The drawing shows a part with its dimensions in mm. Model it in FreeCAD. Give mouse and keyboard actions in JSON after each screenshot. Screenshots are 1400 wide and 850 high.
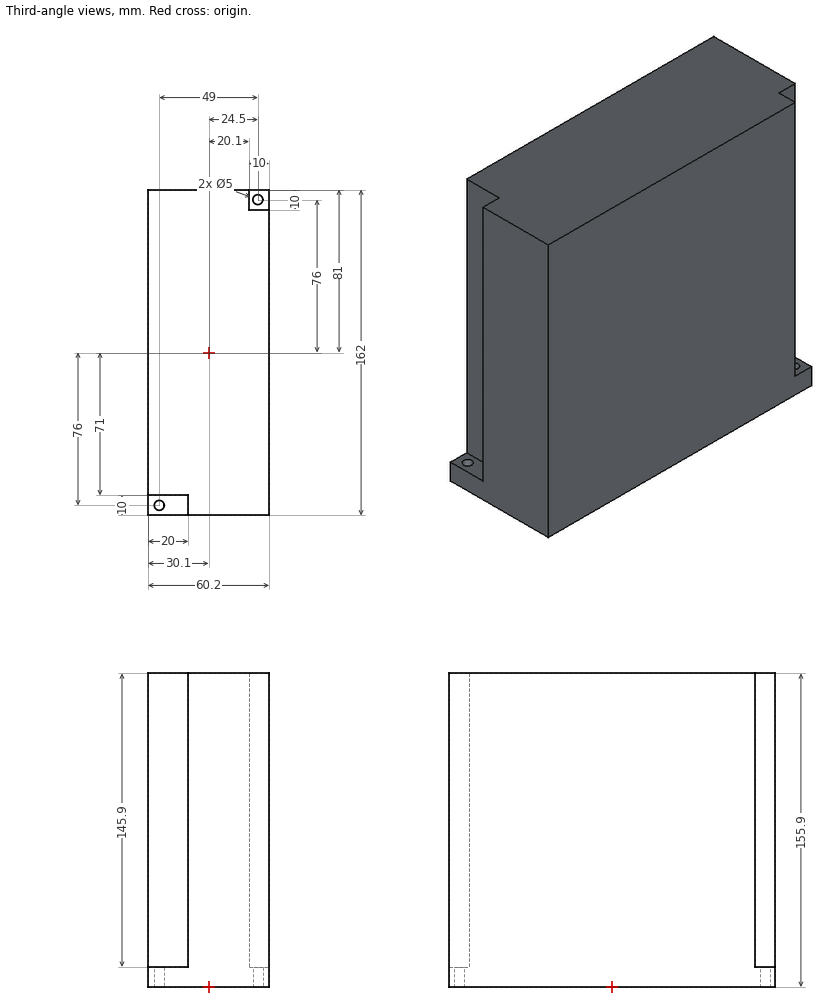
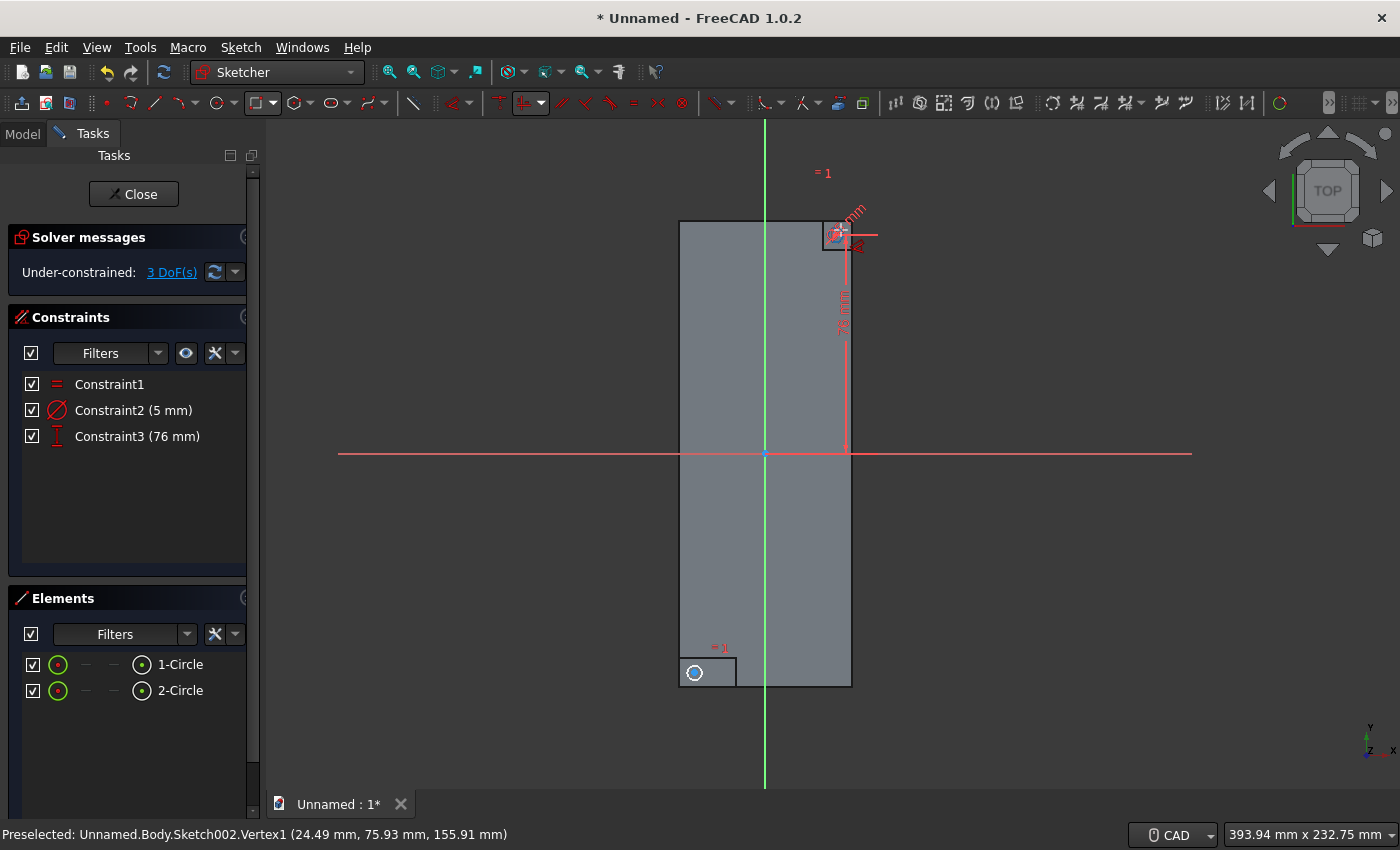
{"action": "left_click", "coordinate": [695, 673]}
{"action": "left_click", "coordinate": [661, 563]}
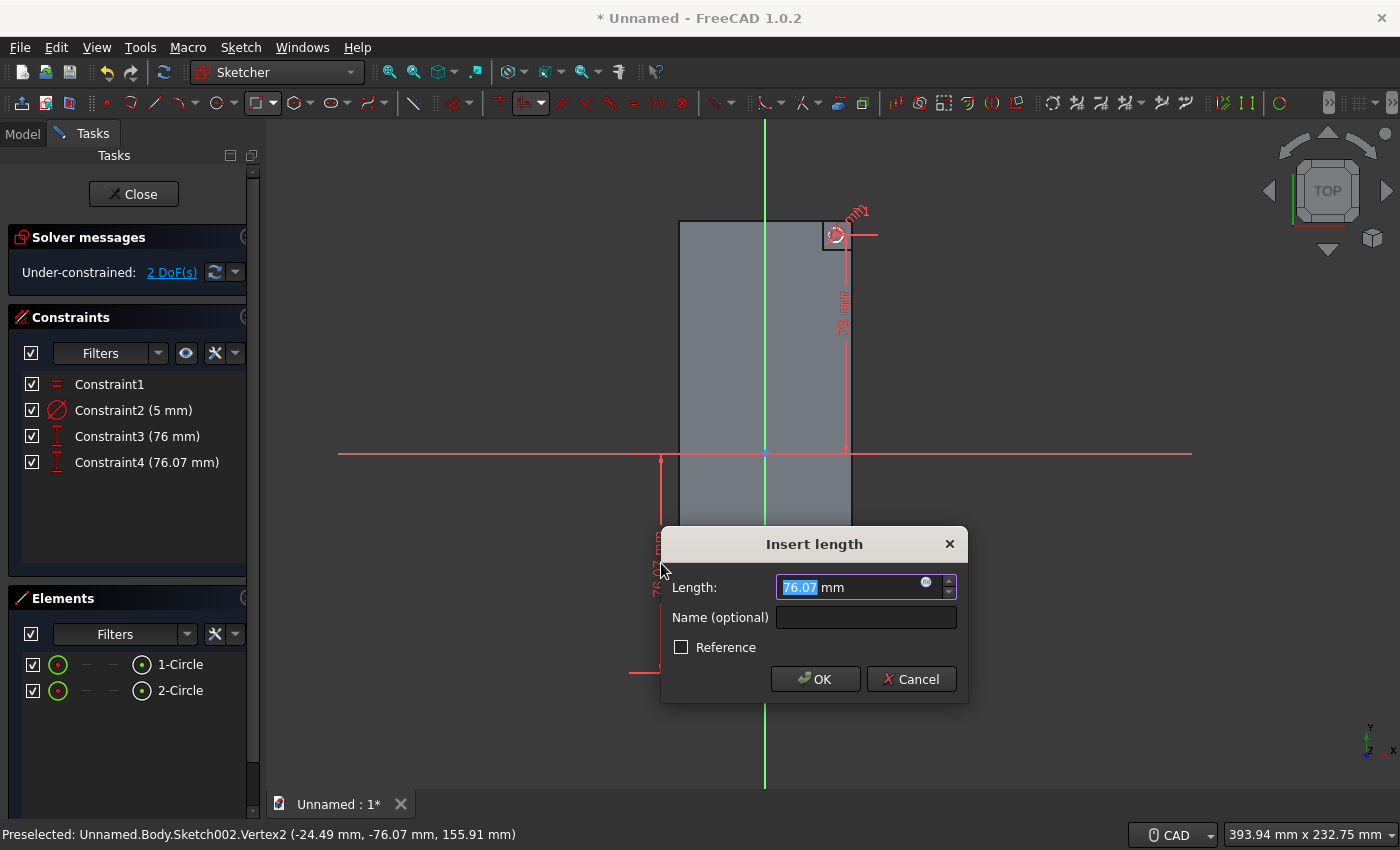
{"action": "type", "text": "76"}
{"action": "key", "text": "Return"}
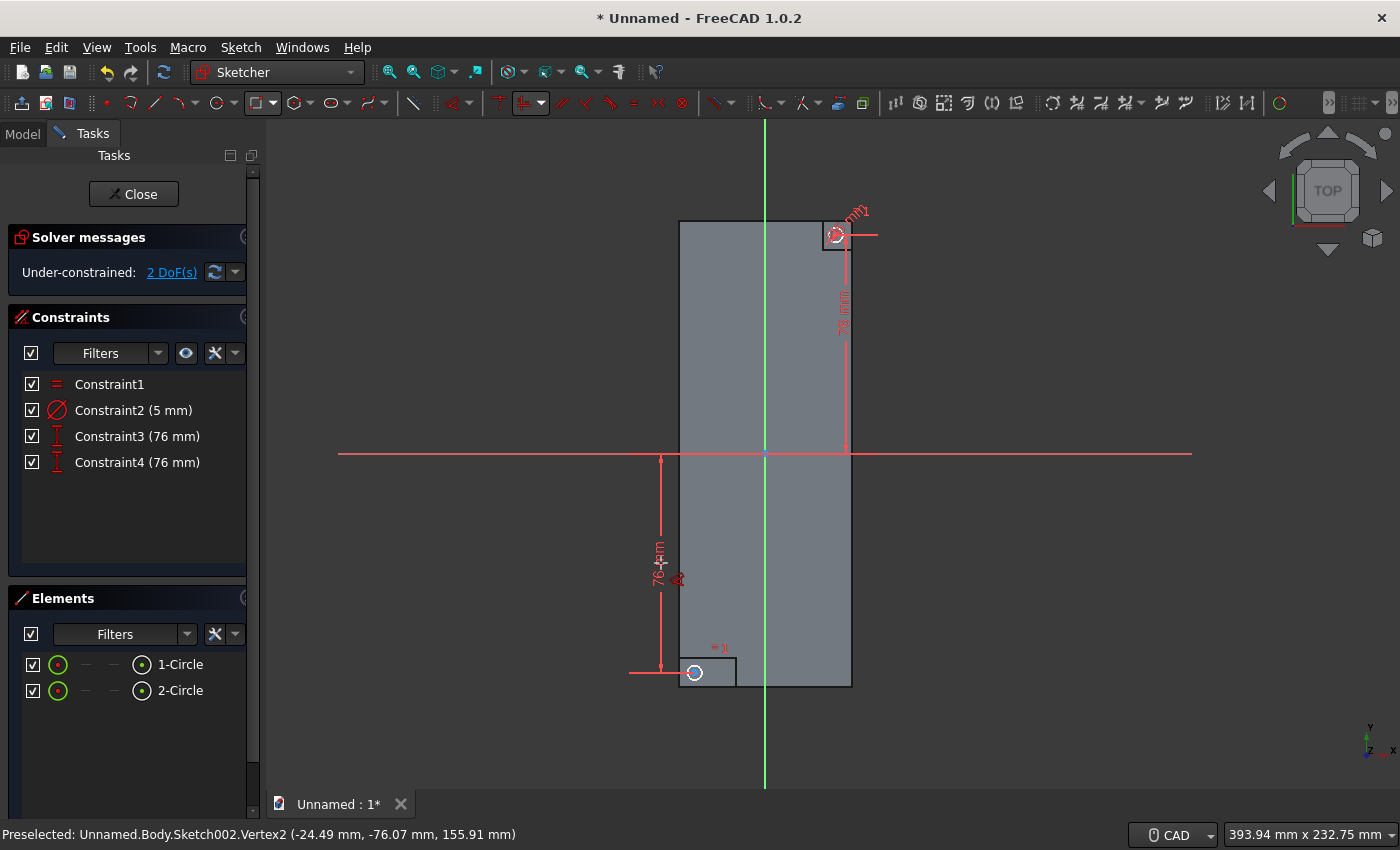
{"action": "left_click", "coordinate": [836, 235]}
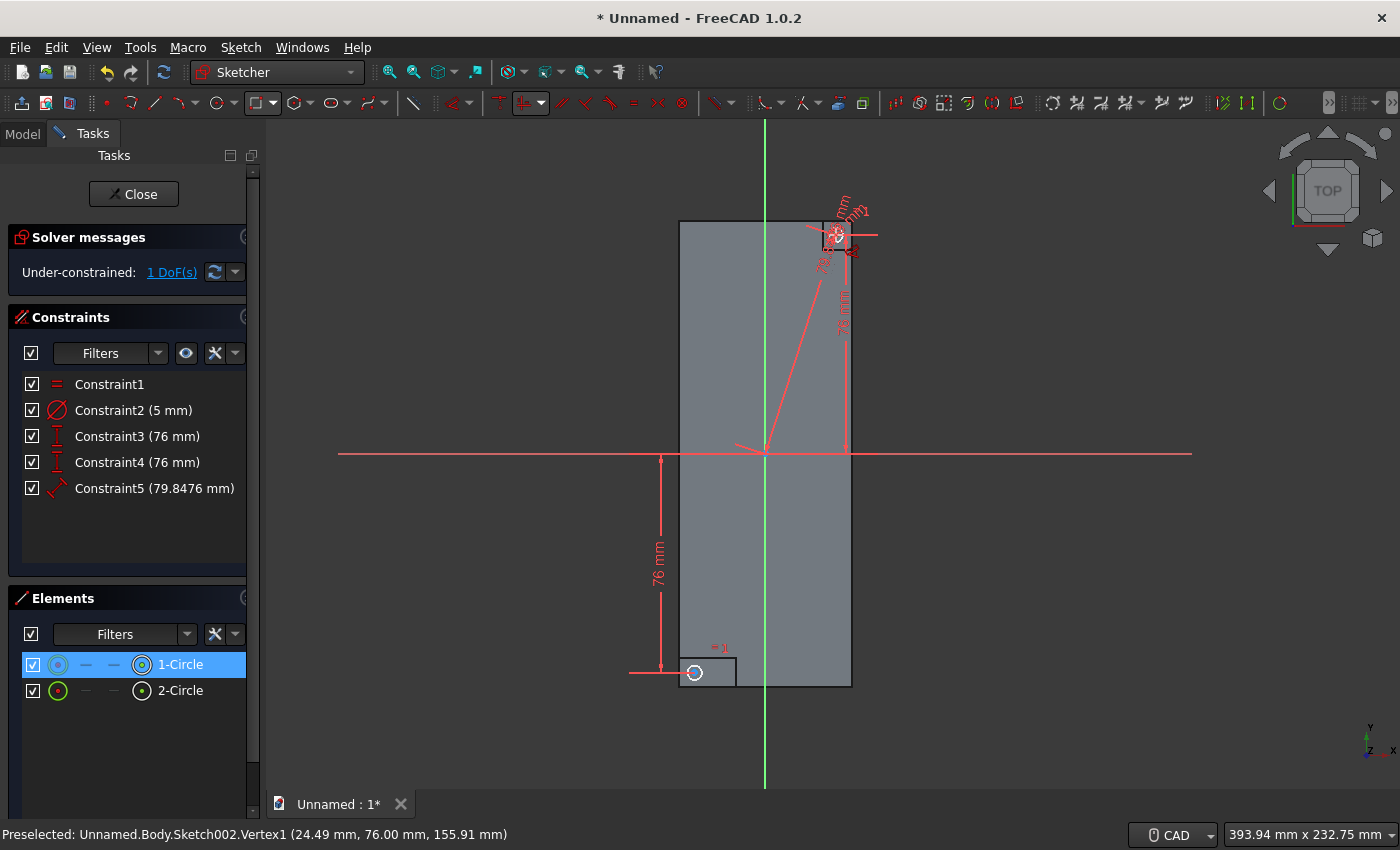
{"action": "left_click", "coordinate": [695, 673]}
{"action": "left_click", "coordinate": [733, 707]}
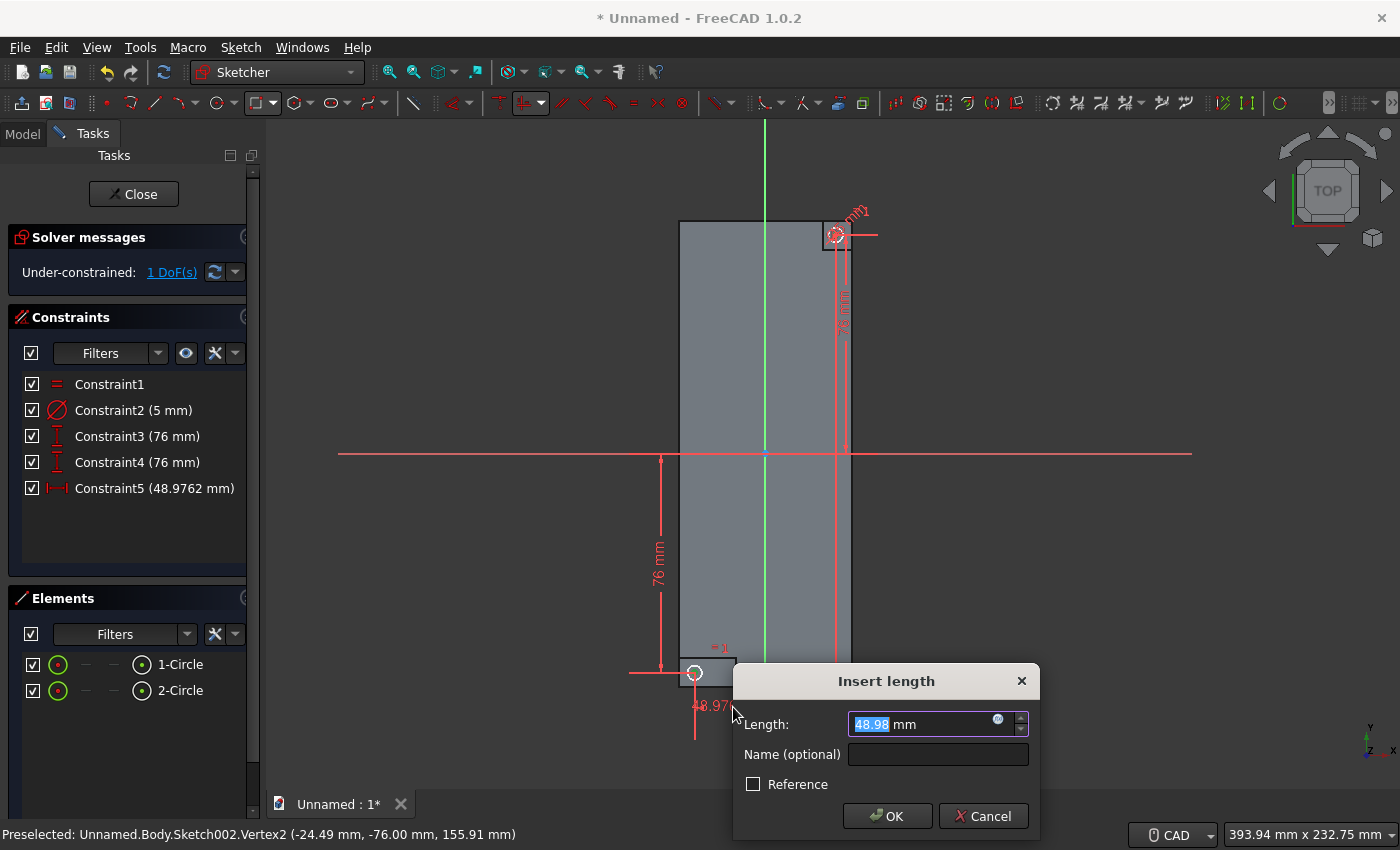
{"action": "type", "text": "49"}
{"action": "key", "text": "Return"}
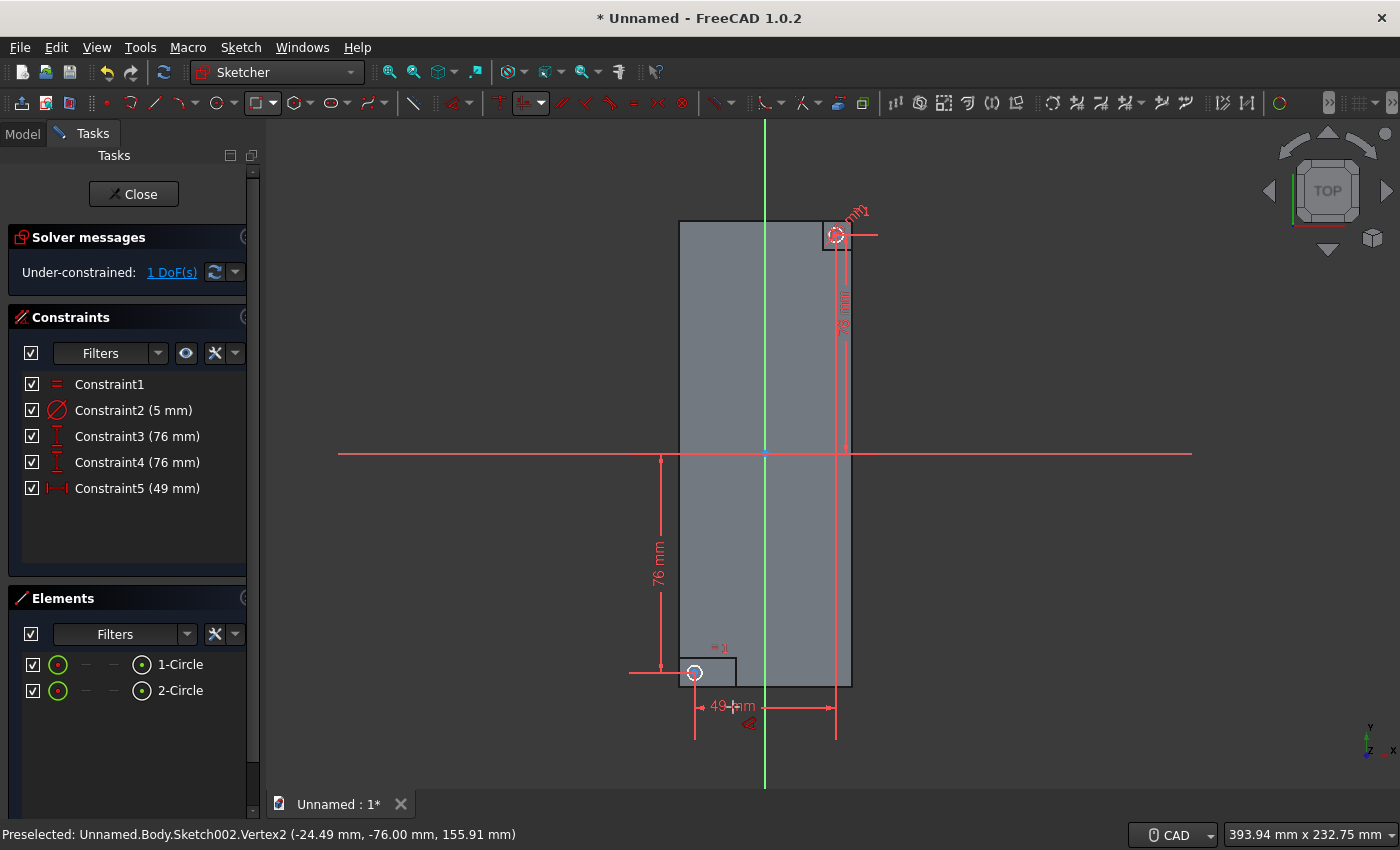
{"action": "left_click", "coordinate": [836, 235]}
{"action": "left_click", "coordinate": [800, 201]}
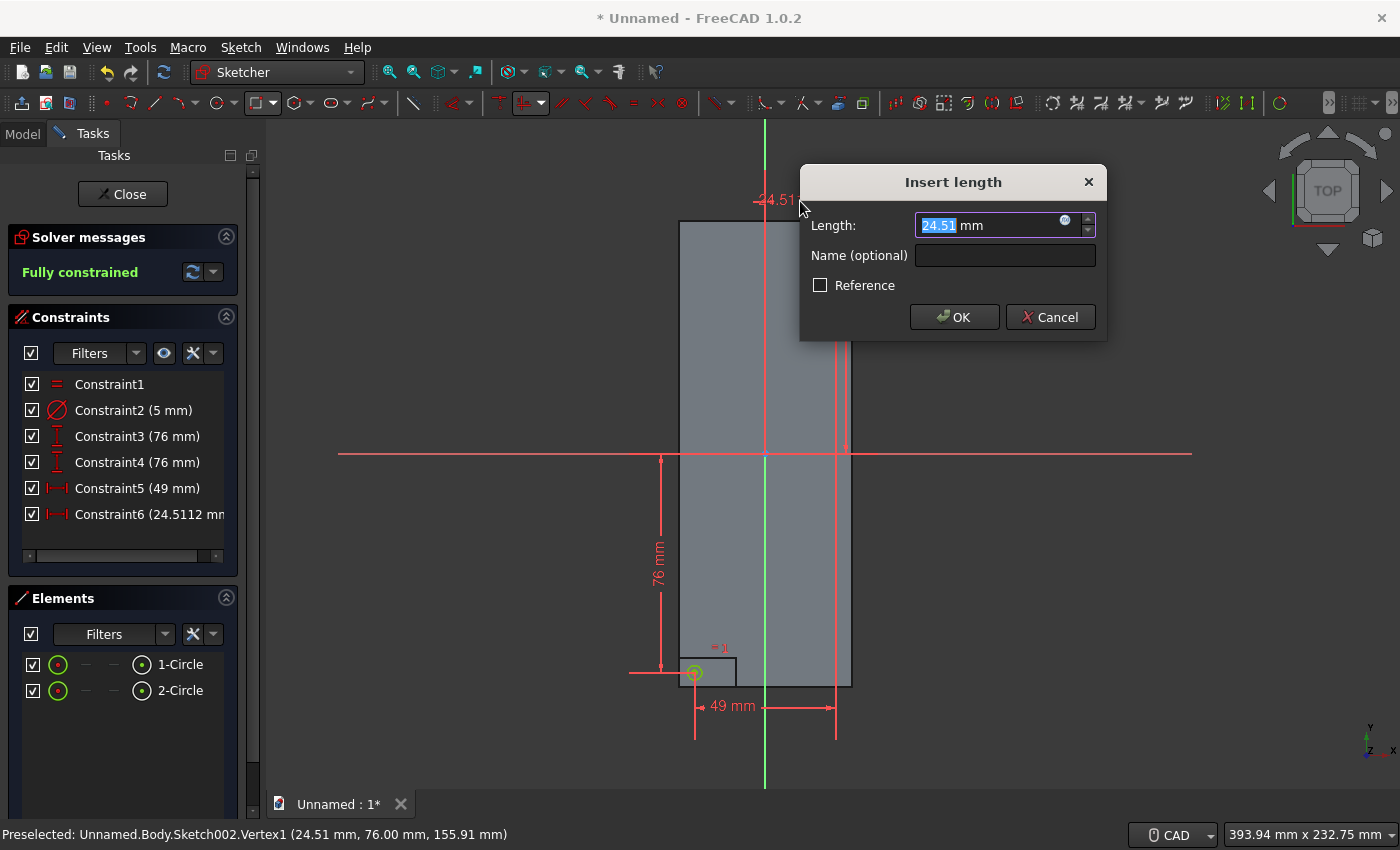
{"action": "type", "text": "24.5"}
{"action": "key", "text": "Return"}
{"action": "key", "text": "Escape"}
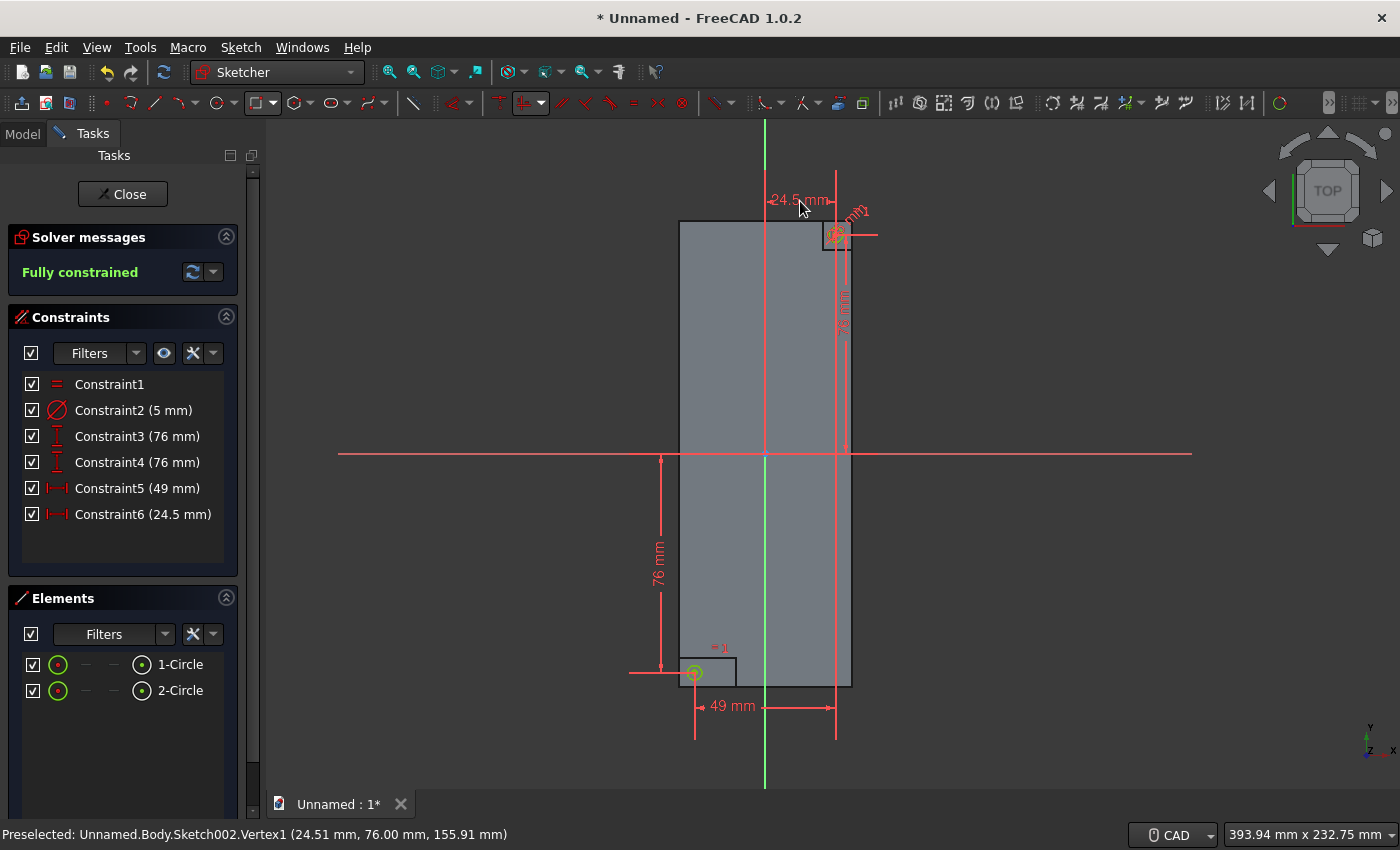
{"action": "left_click", "coordinate": [123, 194]}